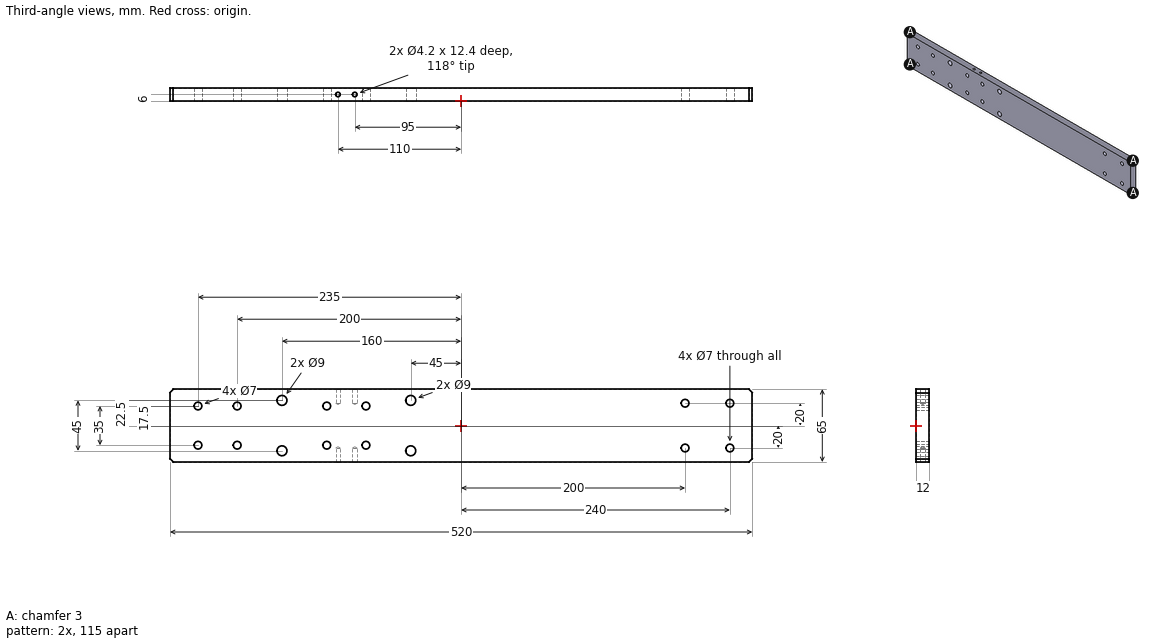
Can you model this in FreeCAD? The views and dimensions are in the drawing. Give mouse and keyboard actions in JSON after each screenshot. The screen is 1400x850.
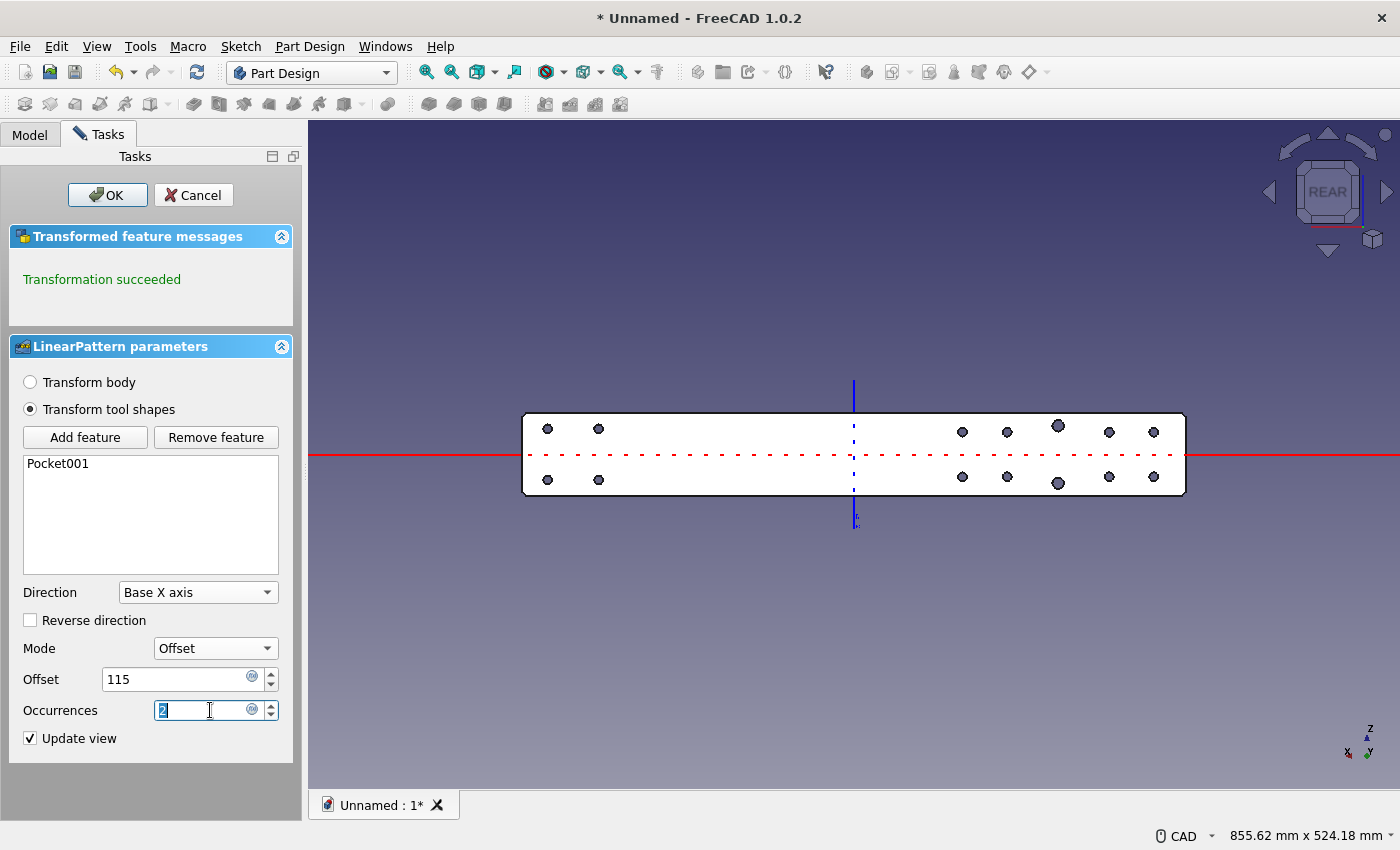
{"action": "type", "text": "2"}
{"action": "key", "text": "Tab"}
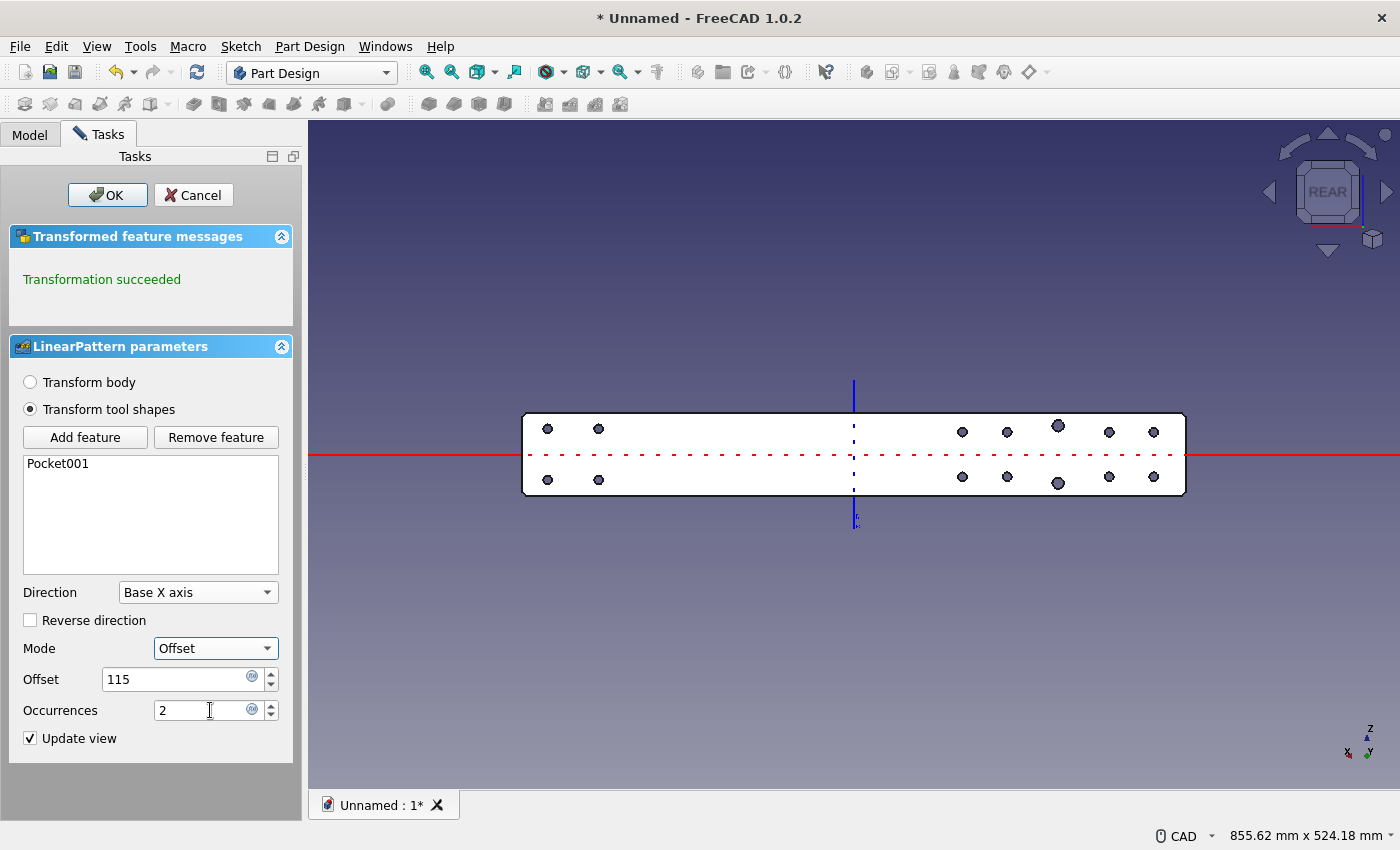
{"action": "left_click", "coordinate": [108, 195]}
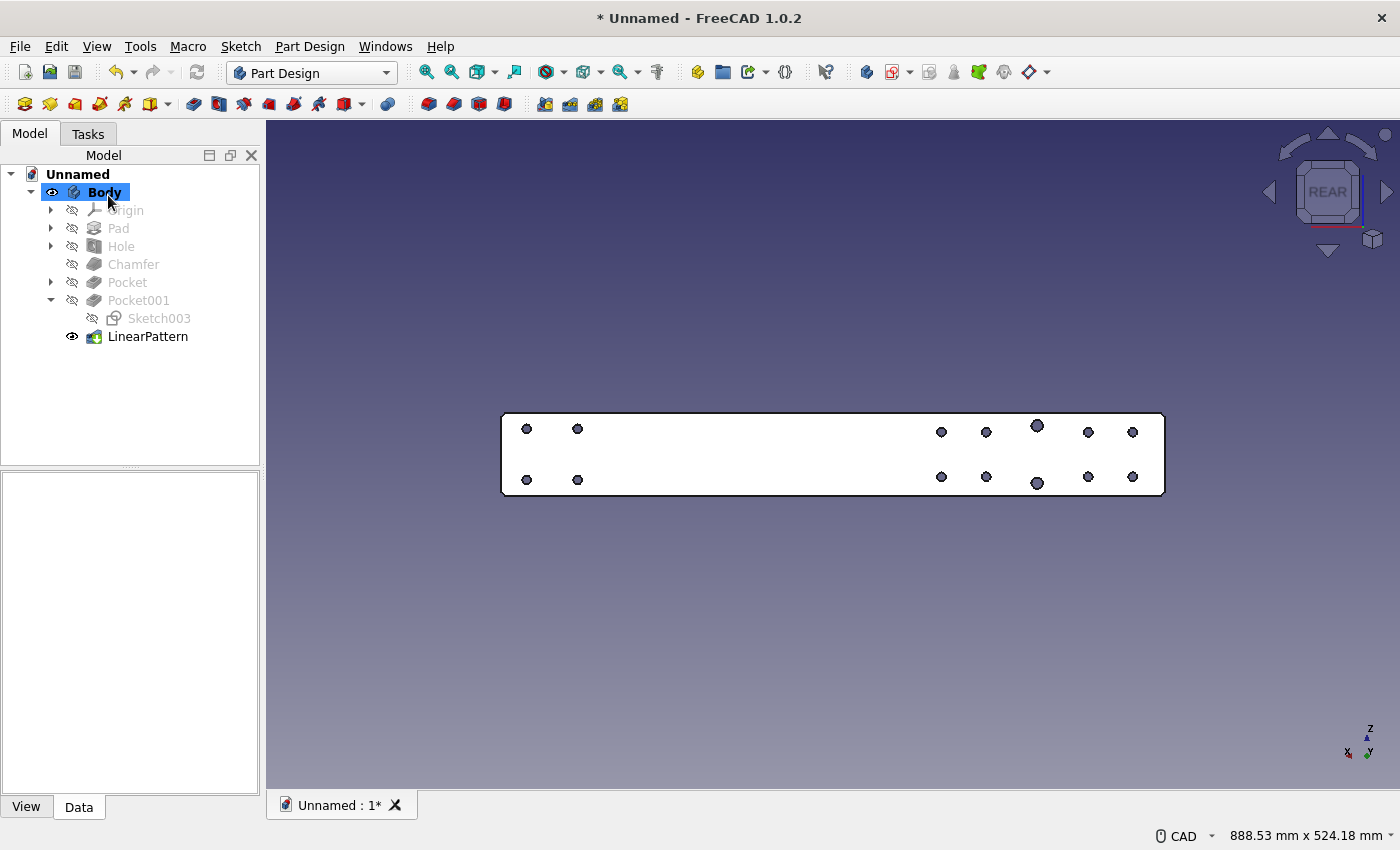
{"action": "left_click", "coordinate": [643, 454]}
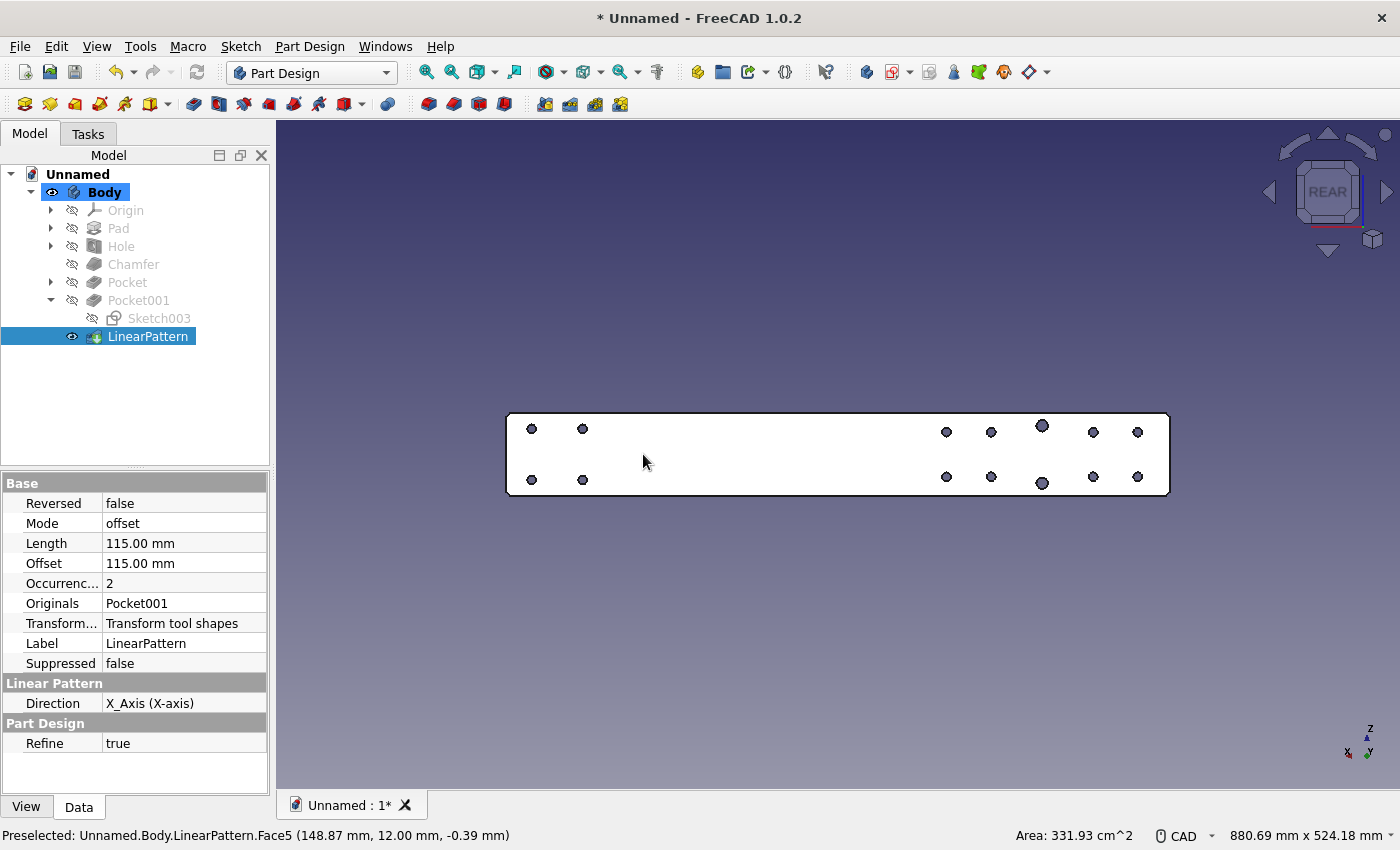
{"action": "left_click", "coordinate": [892, 72]}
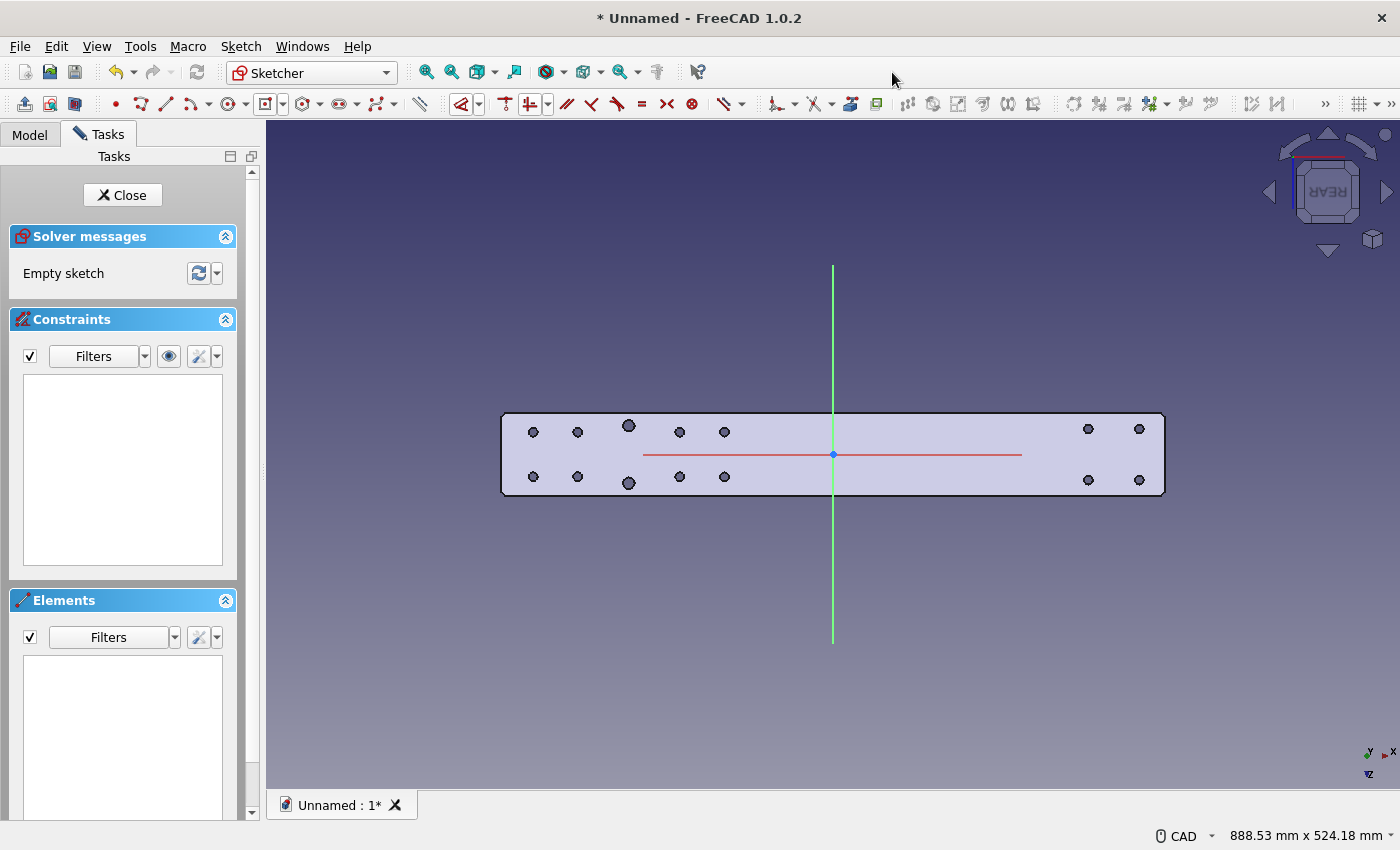
{"action": "scroll", "coordinate": [809, 454], "scroll_direction": "up", "scroll_amount": 9}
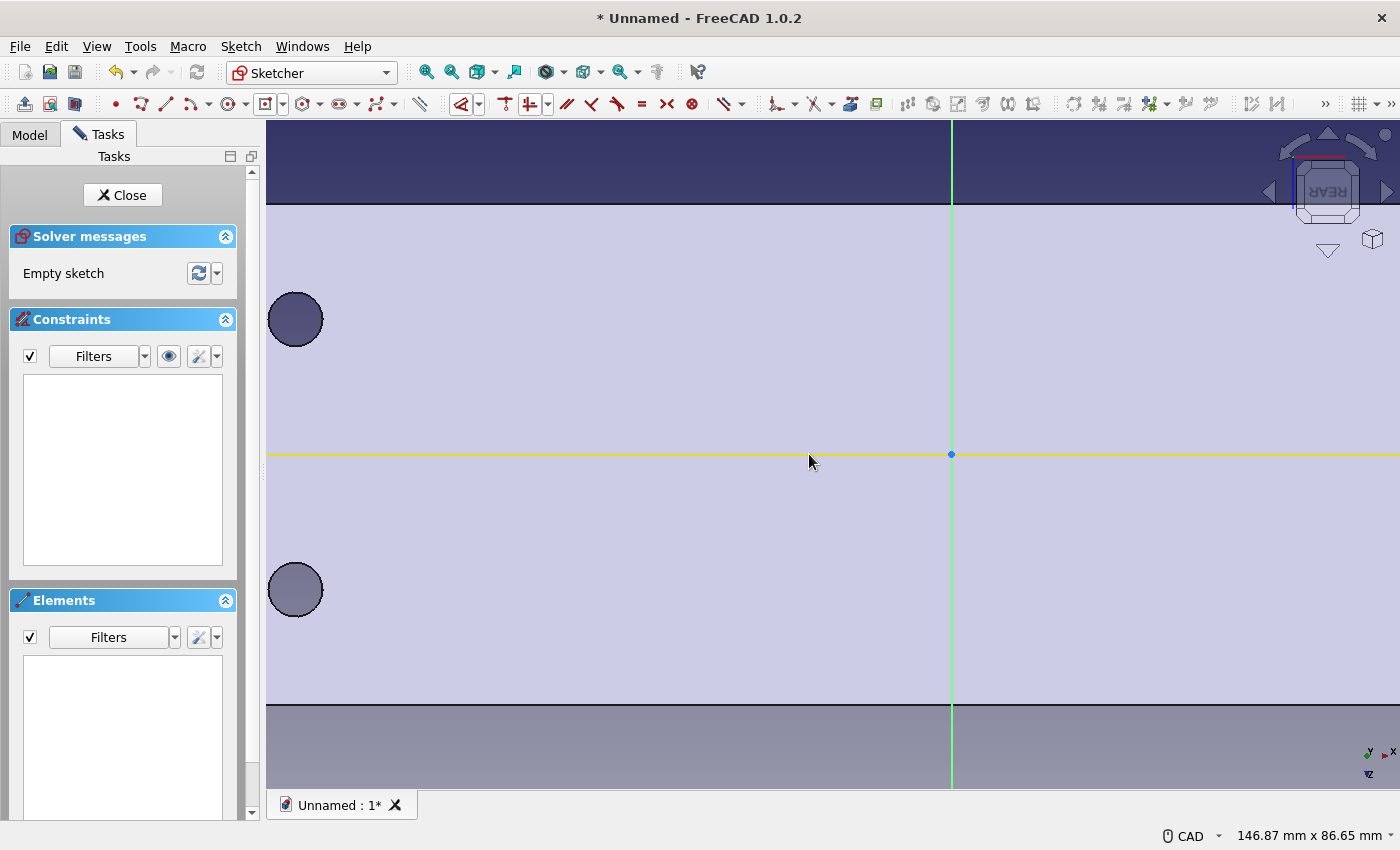
{"action": "left_click", "coordinate": [228, 104]}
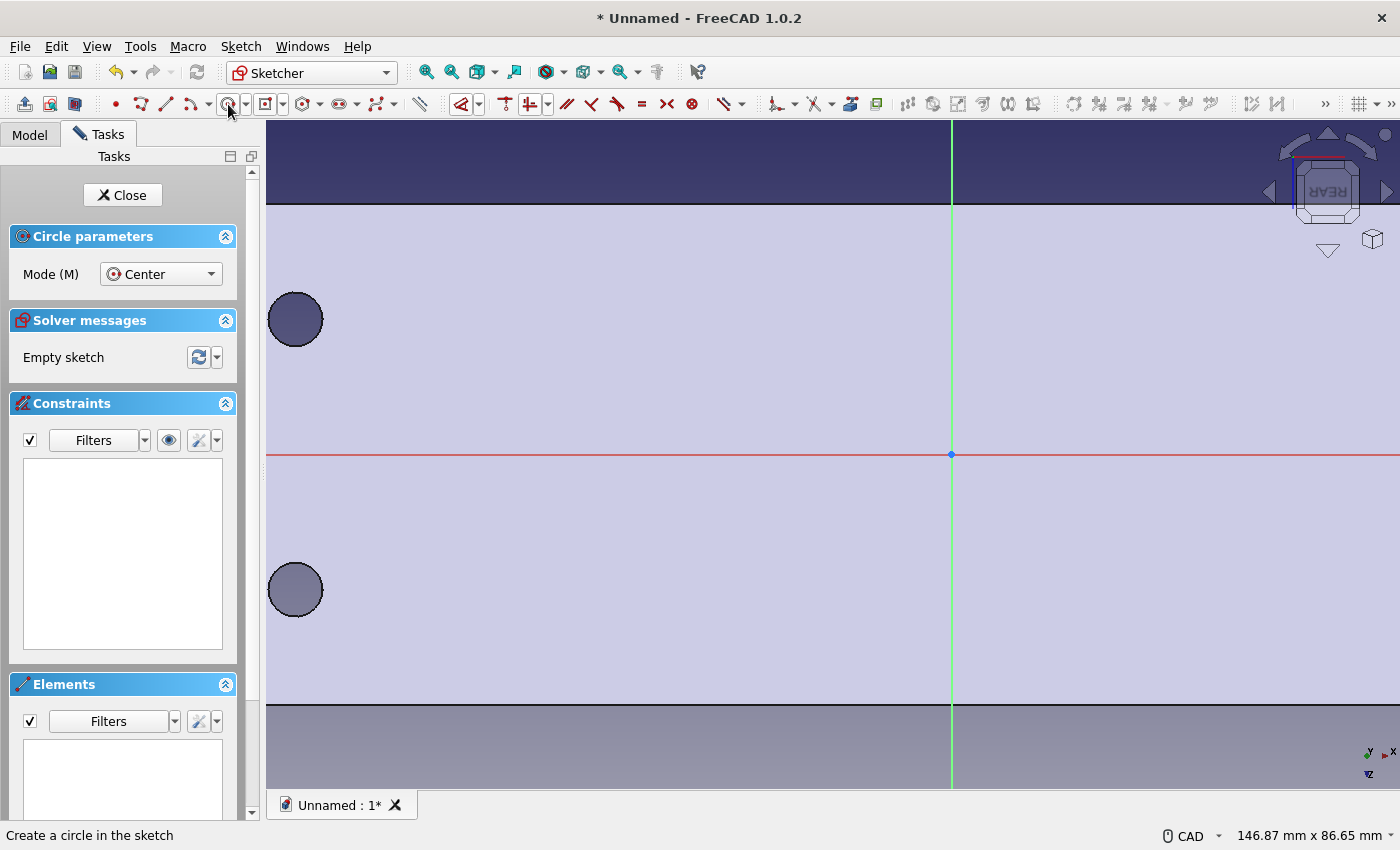
{"action": "left_click", "coordinate": [604, 628]}
{"action": "left_click", "coordinate": [629, 604]}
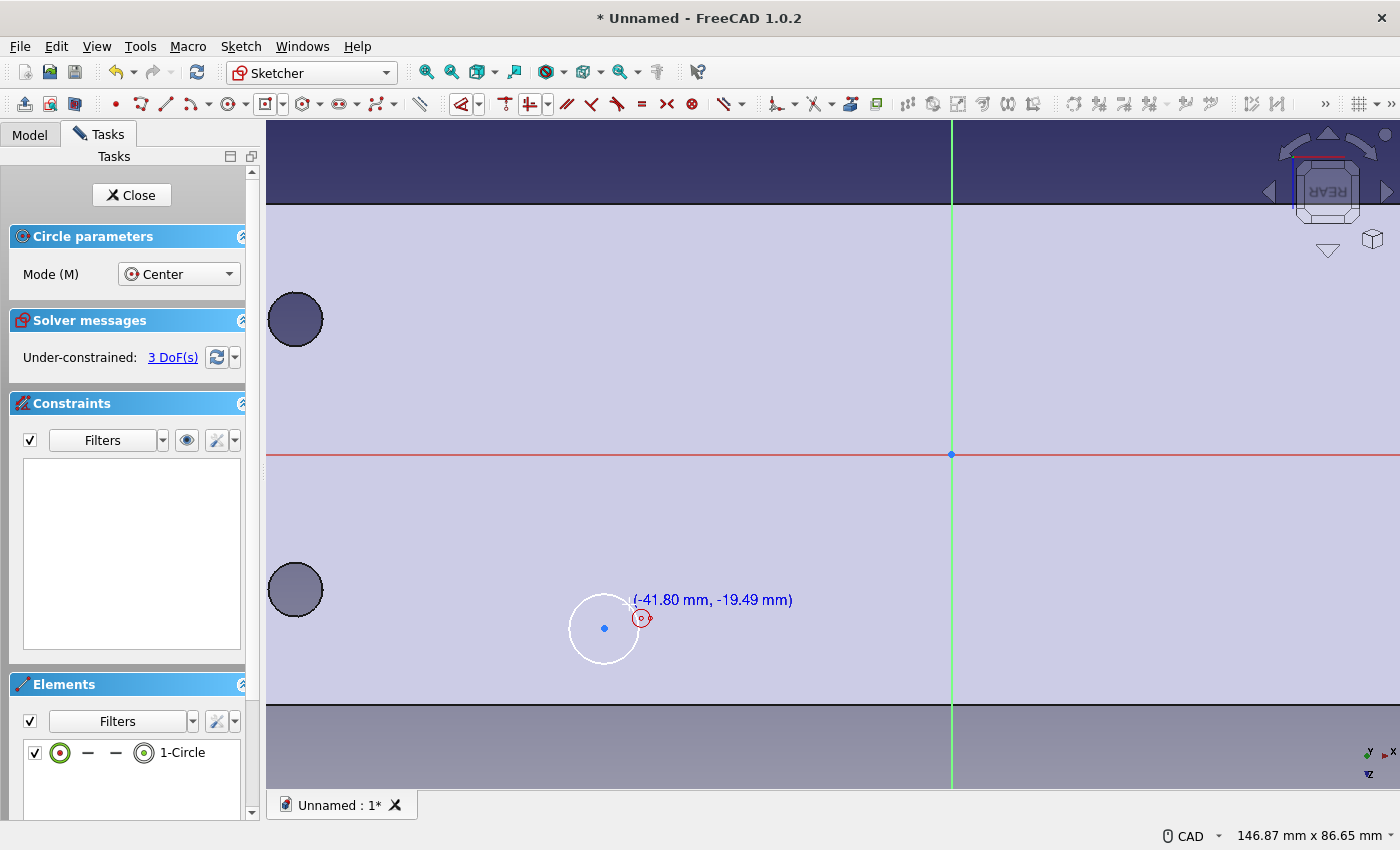
{"action": "left_click", "coordinate": [604, 281]}
{"action": "left_click", "coordinate": [629, 256]}
{"action": "key", "text": "Escape"}